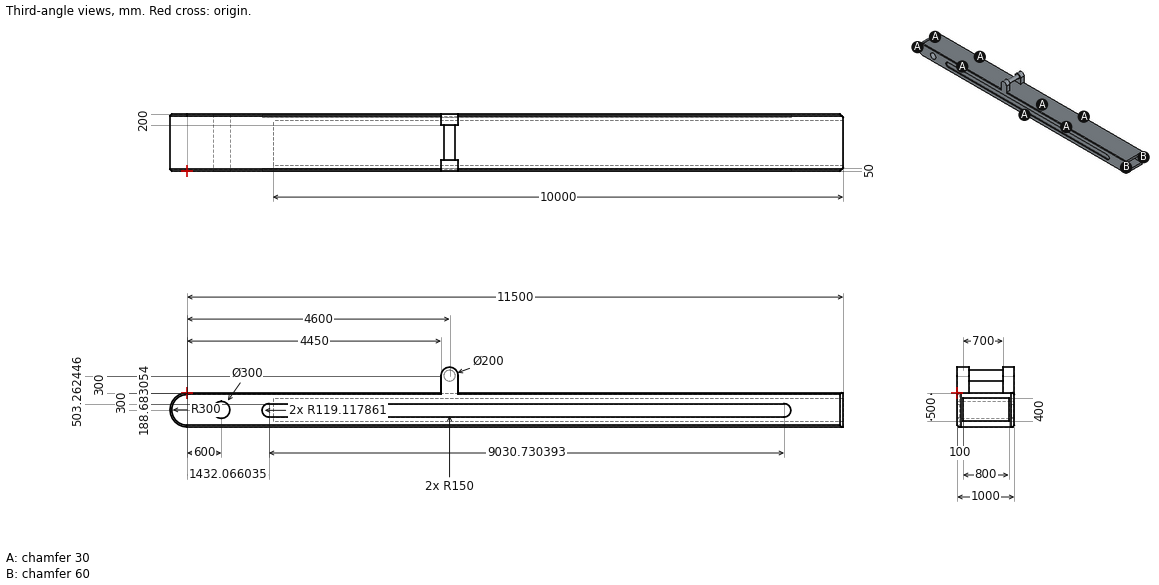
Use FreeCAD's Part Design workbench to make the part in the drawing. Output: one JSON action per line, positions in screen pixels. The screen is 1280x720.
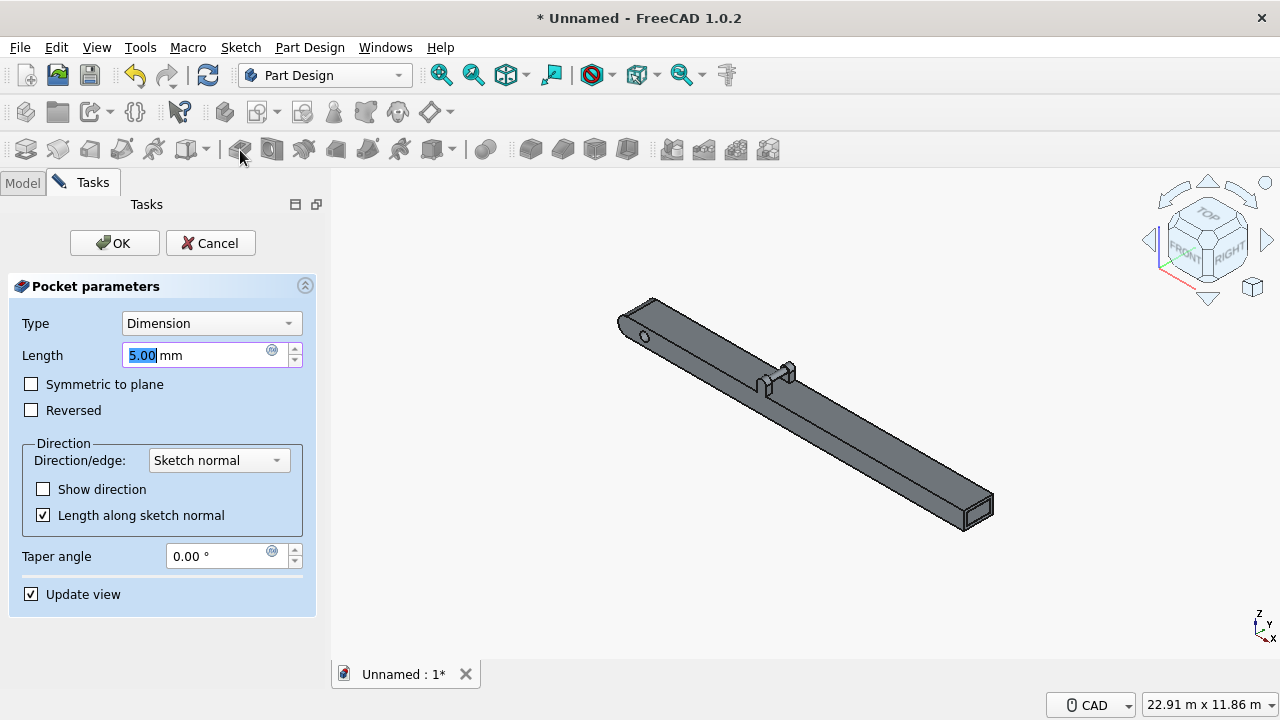
{"action": "type", "text": "10000"}
{"action": "key", "text": "Tab"}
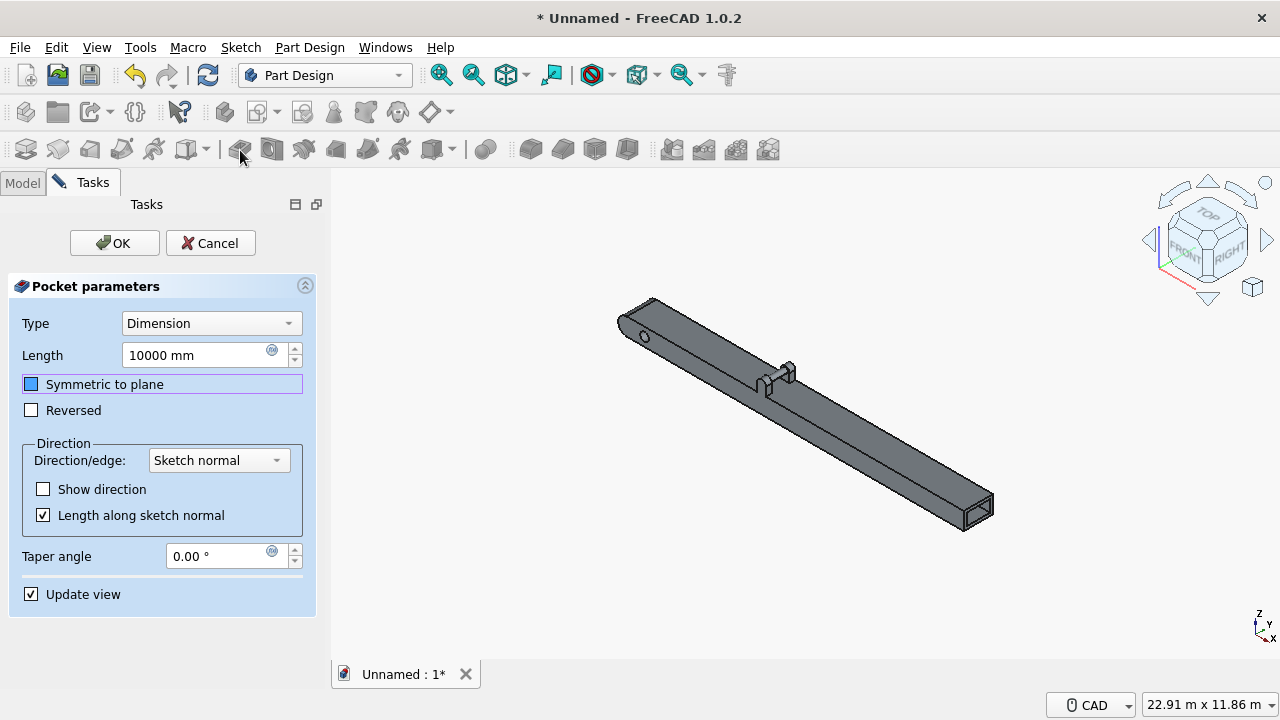
{"action": "left_click", "coordinate": [115, 243]}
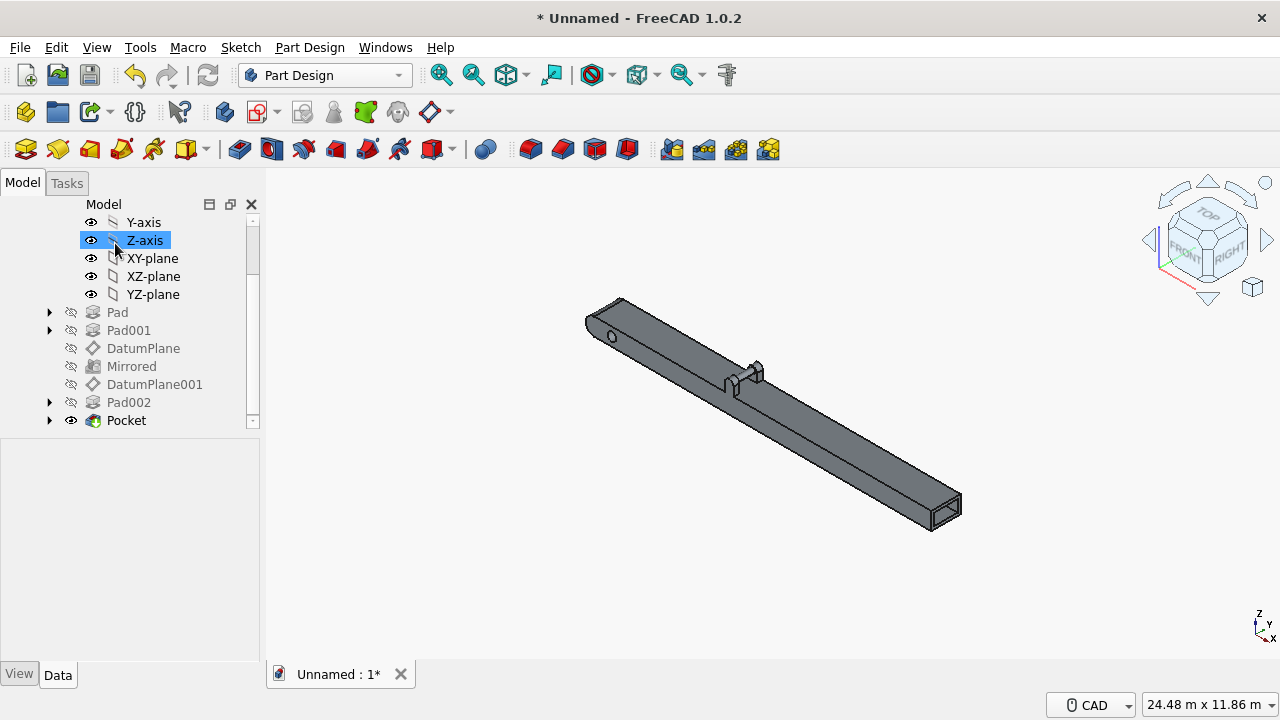
{"action": "left_click", "coordinate": [258, 112]}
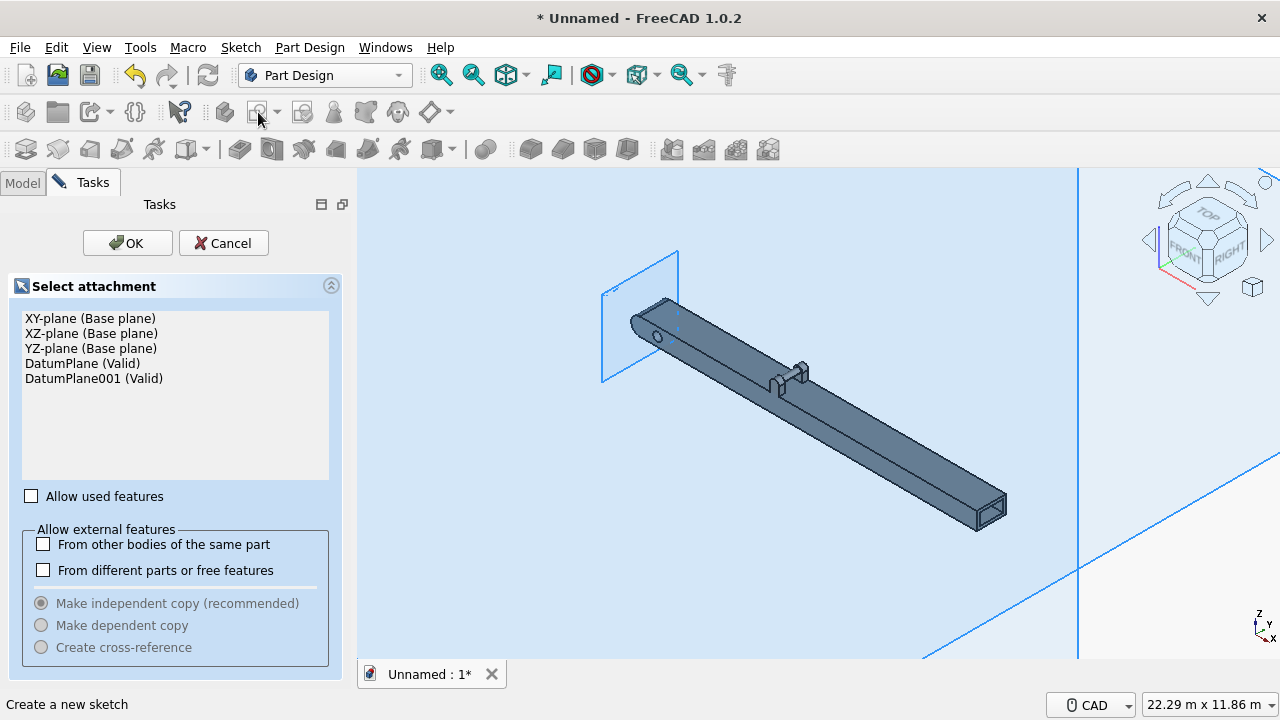
{"action": "left_click", "coordinate": [82, 334]}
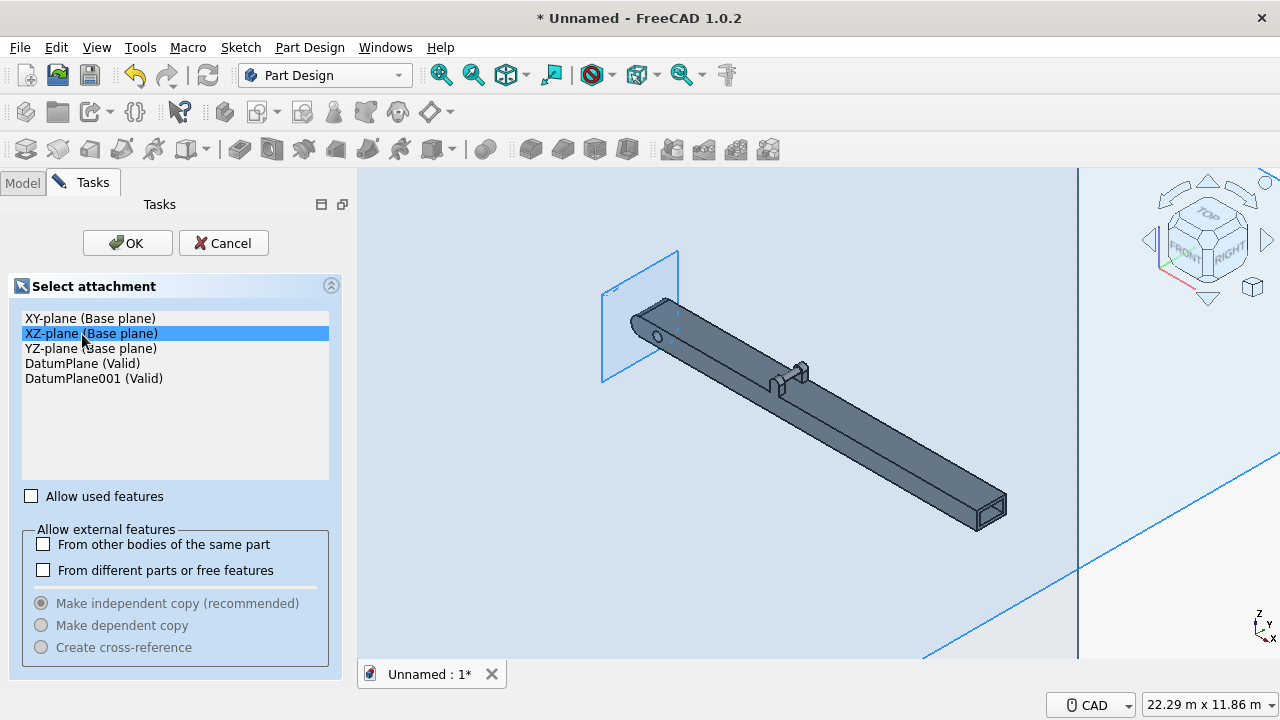
{"action": "left_click", "coordinate": [128, 243]}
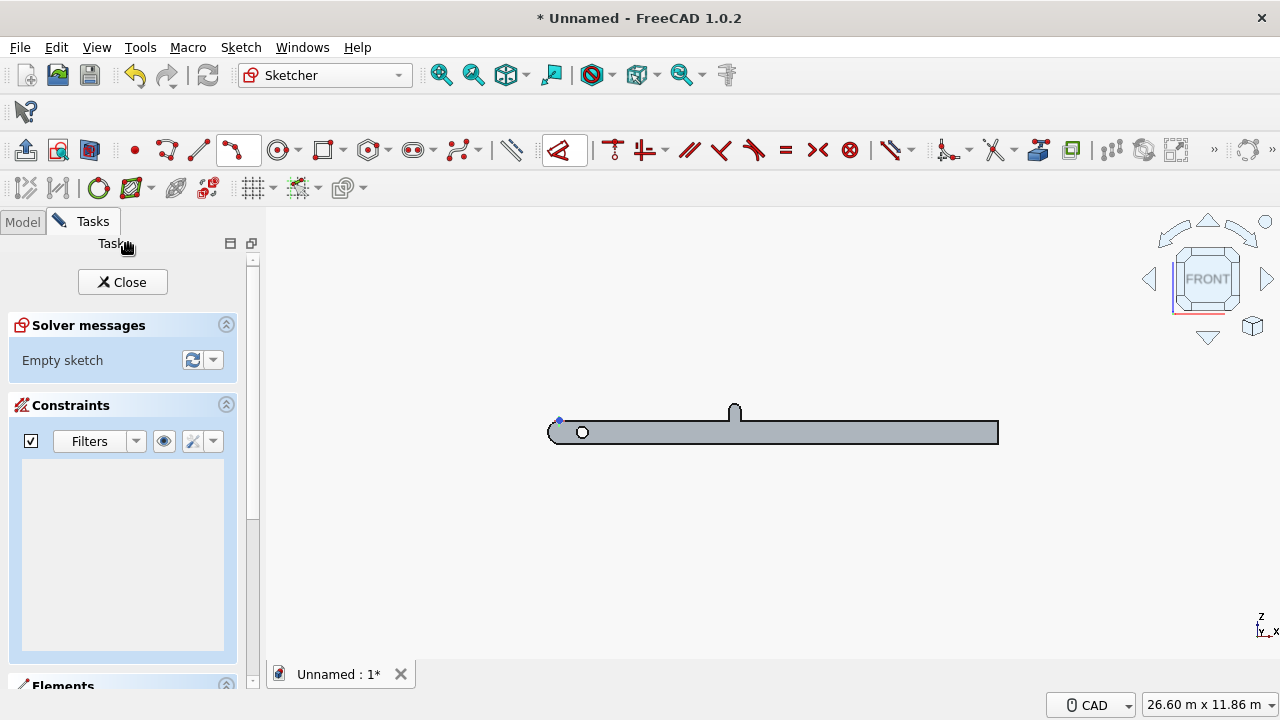
{"action": "scroll", "coordinate": [876, 421], "scroll_direction": "up", "scroll_amount": 2}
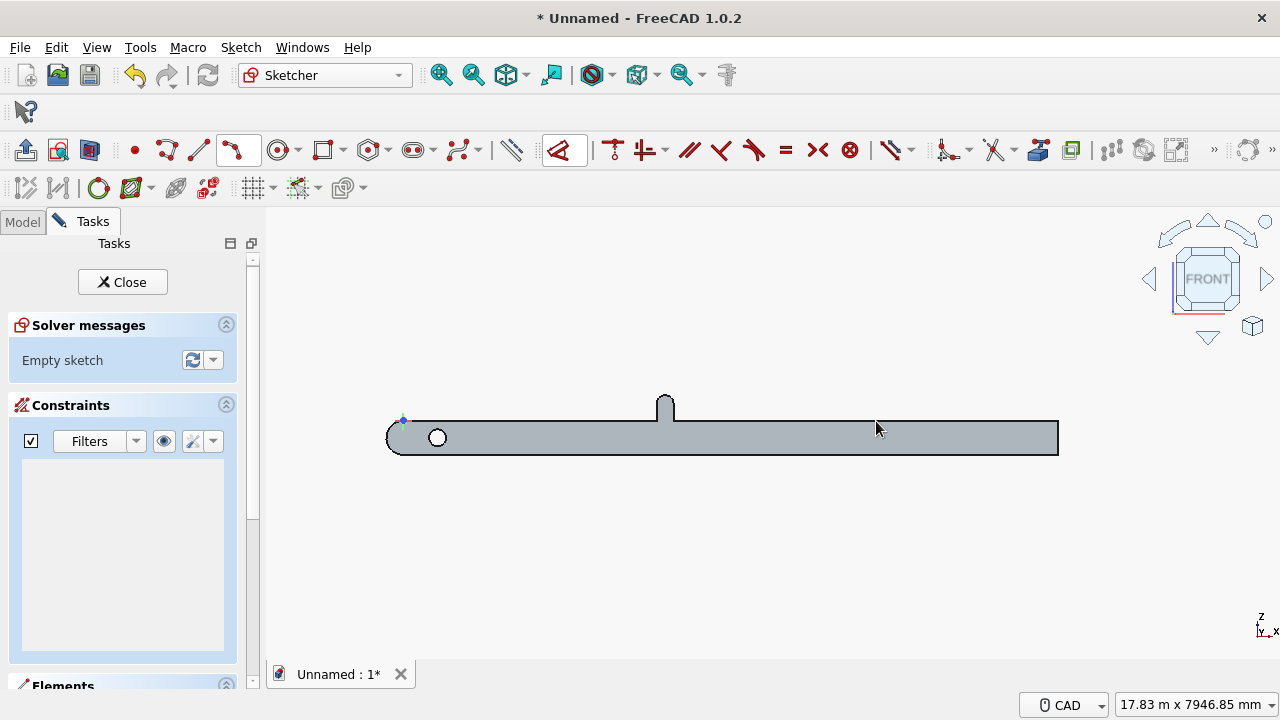
{"action": "left_click", "coordinate": [414, 150]}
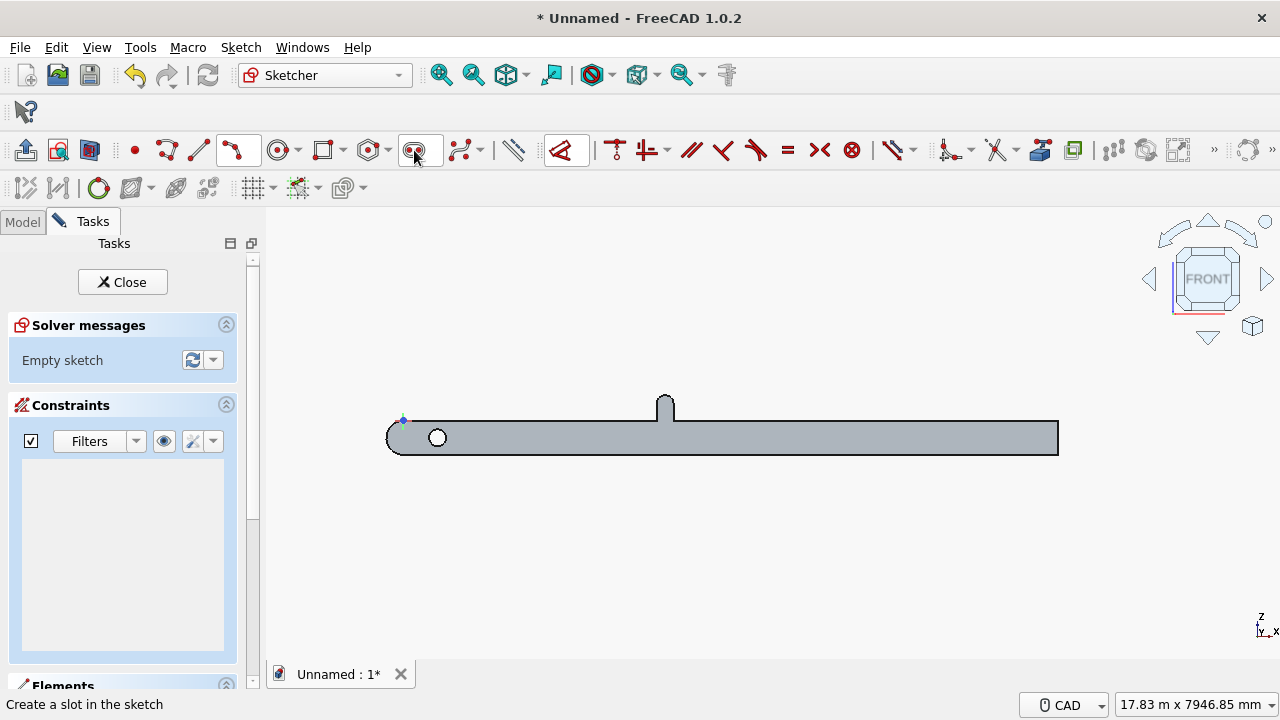
{"action": "scroll", "coordinate": [485, 438], "scroll_direction": "up", "scroll_amount": 7}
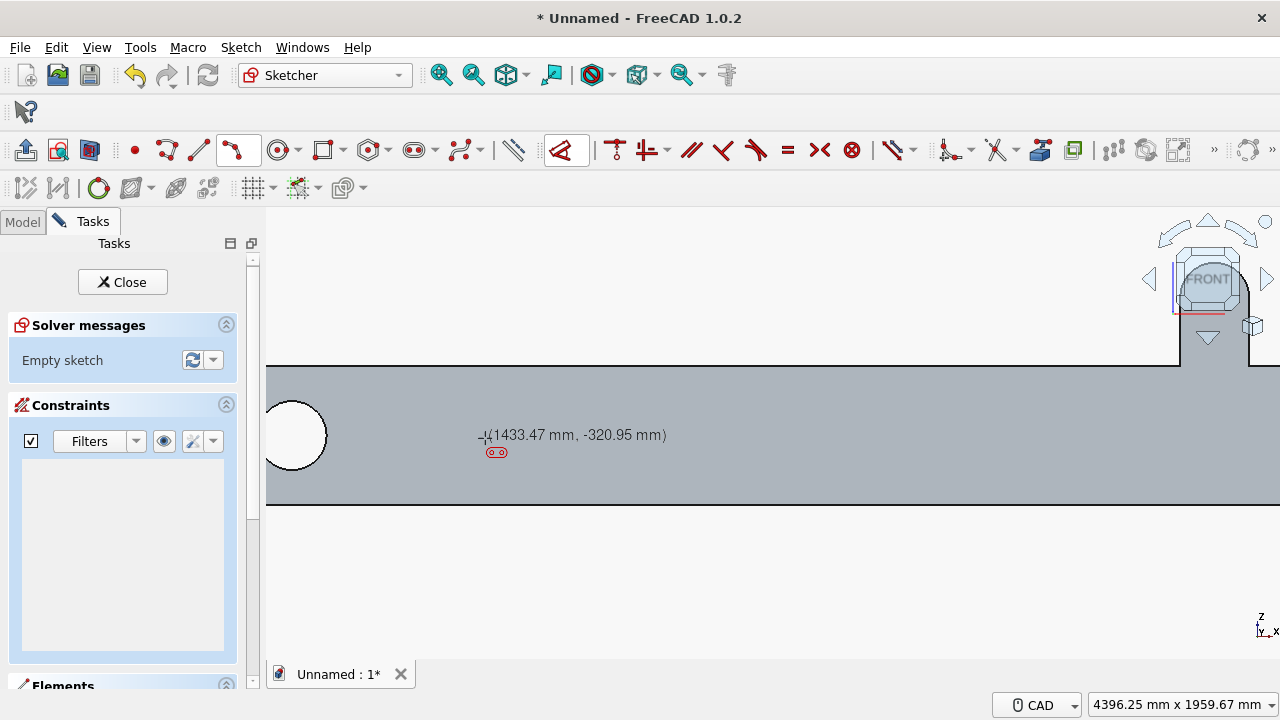
{"action": "scroll", "coordinate": [485, 439], "scroll_direction": "down", "scroll_amount": 7}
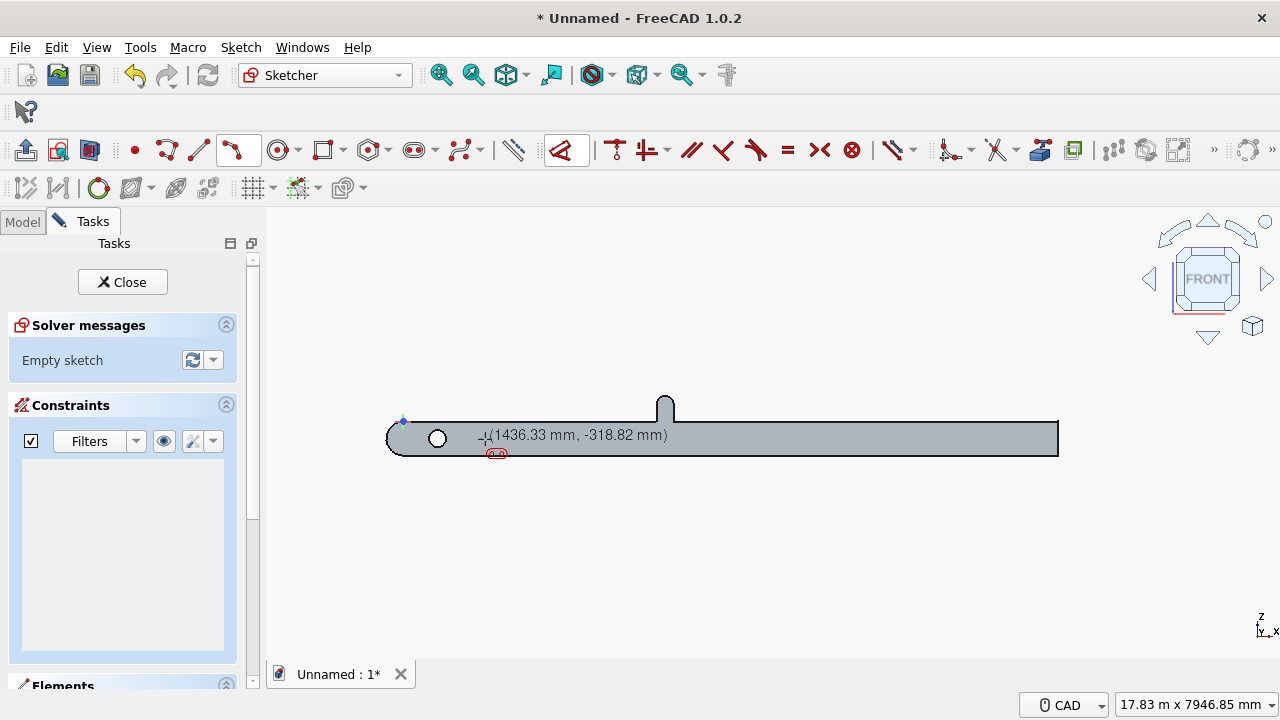
{"action": "left_click", "coordinate": [485, 439]}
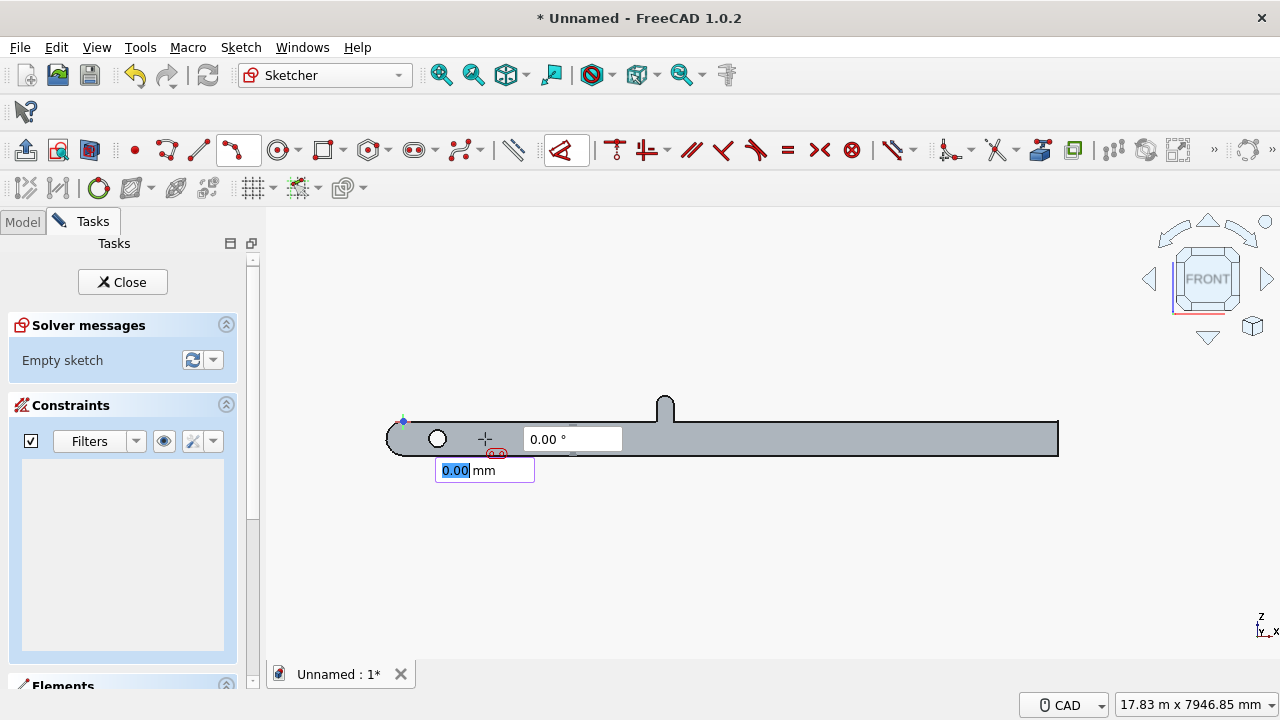
{"action": "left_click", "coordinate": [999, 439]}